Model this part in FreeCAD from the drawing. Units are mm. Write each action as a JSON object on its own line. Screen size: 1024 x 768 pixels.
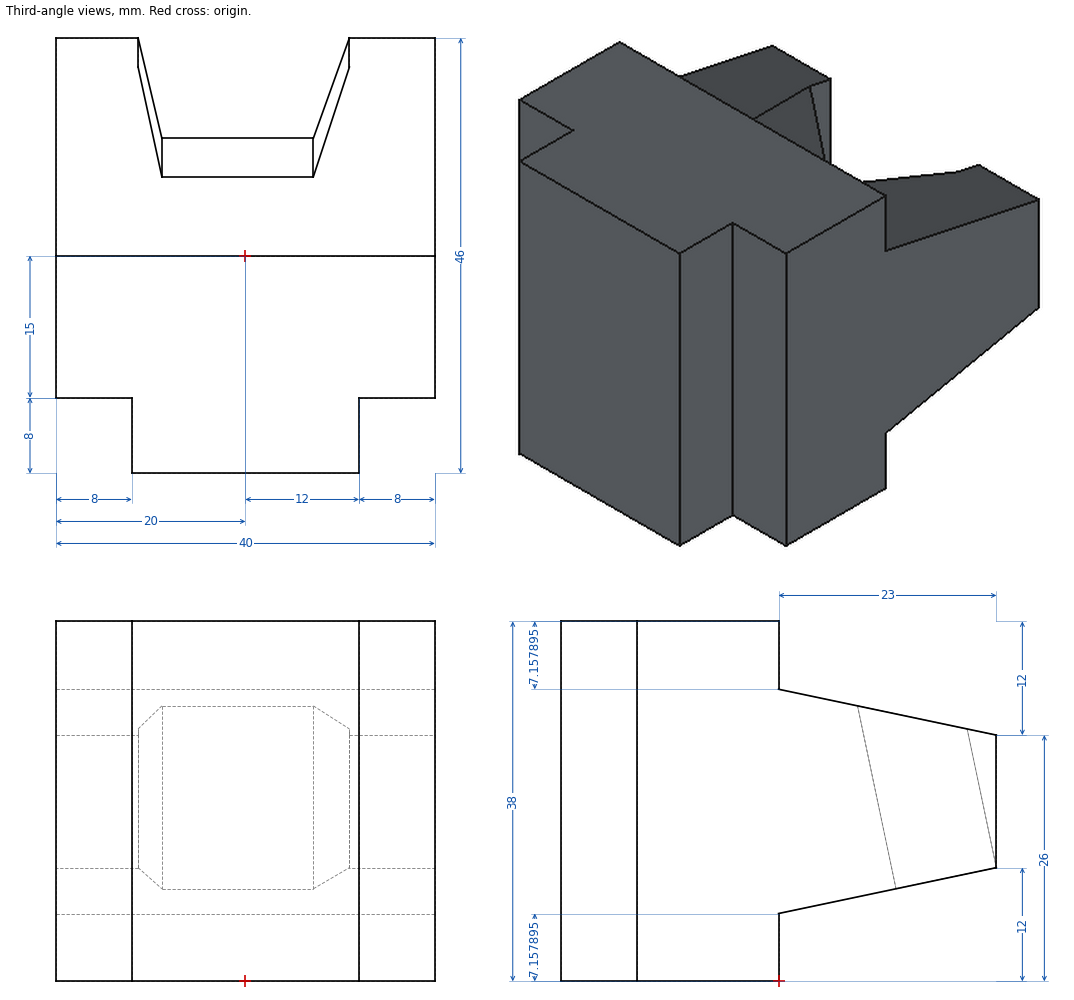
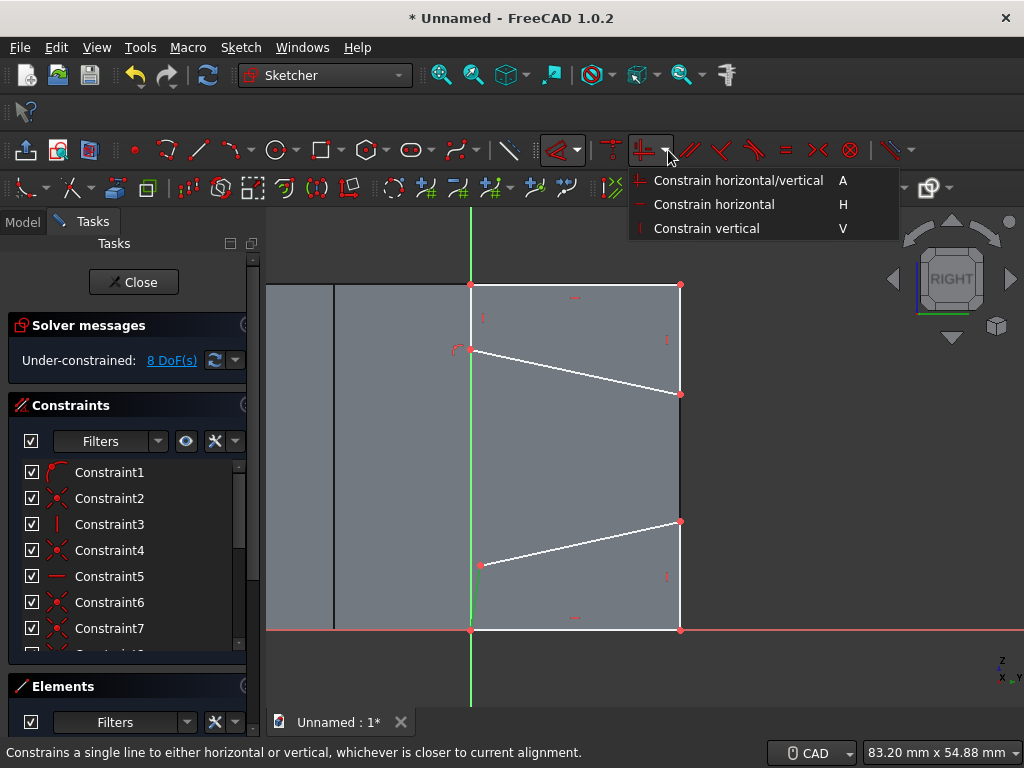
{"action": "left_click", "coordinate": [764, 228]}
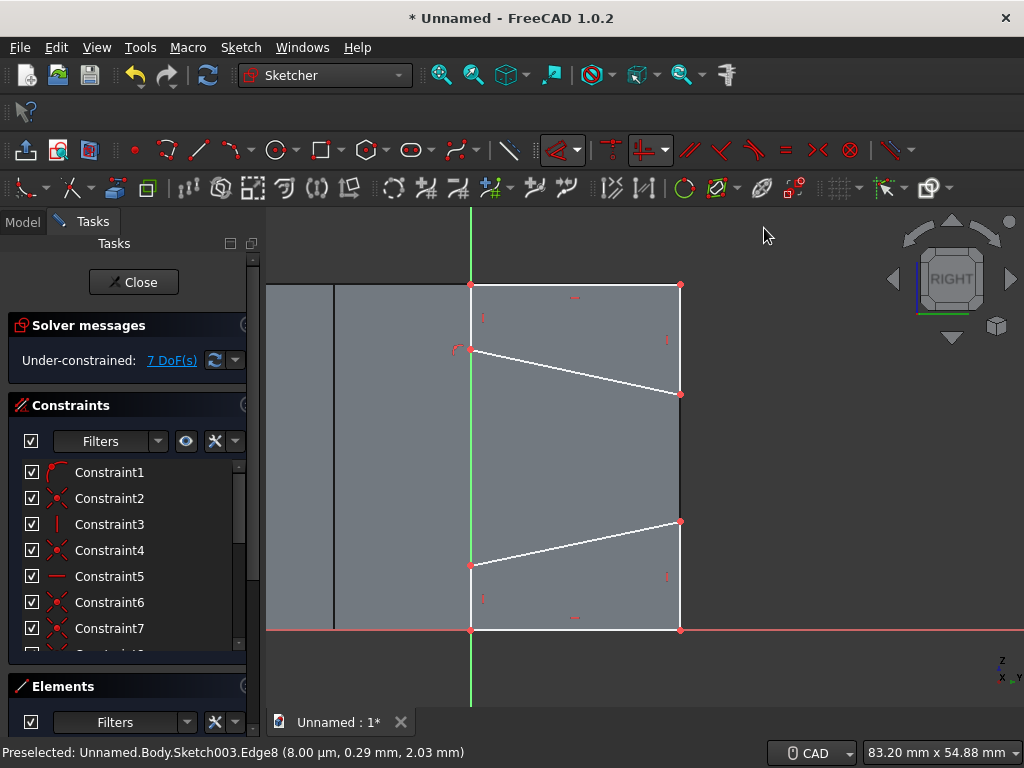
{"action": "left_click", "coordinate": [680, 362]}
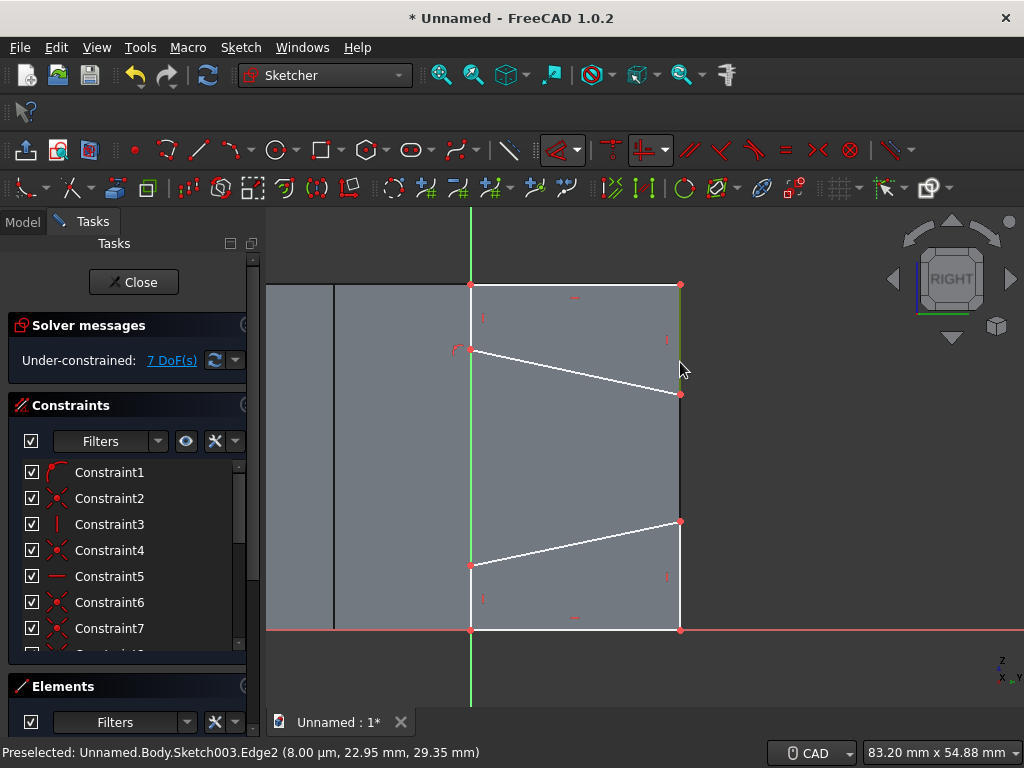
{"action": "key", "text": "i"}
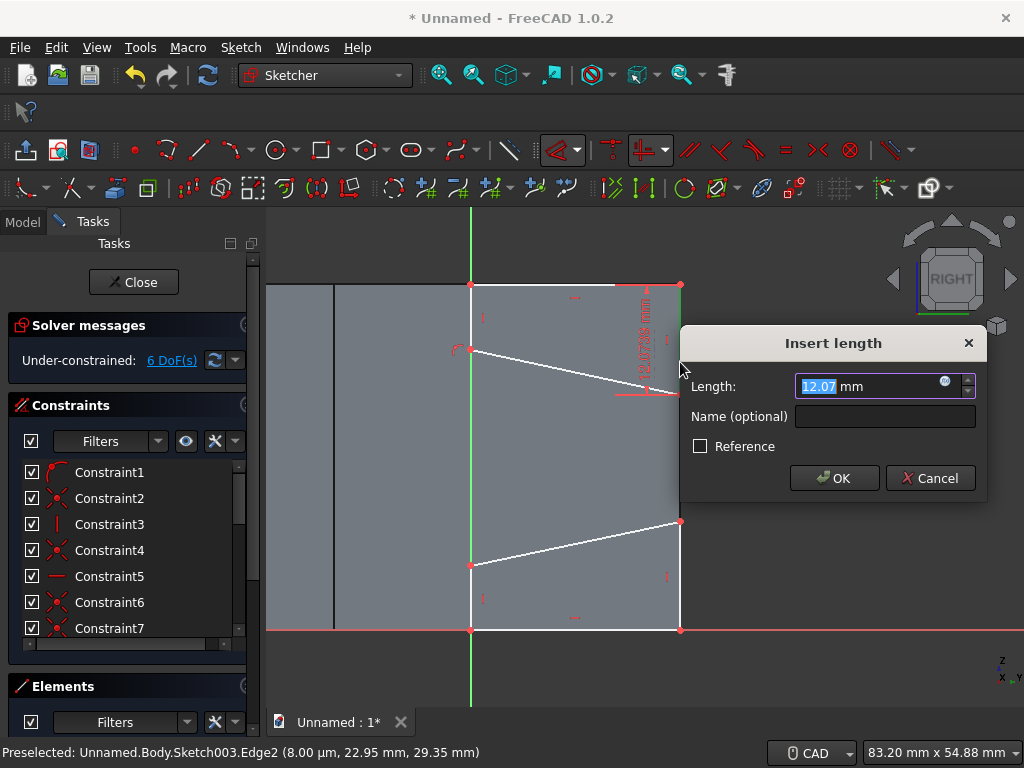
{"action": "type", "text": "12"}
{"action": "key", "text": "Return"}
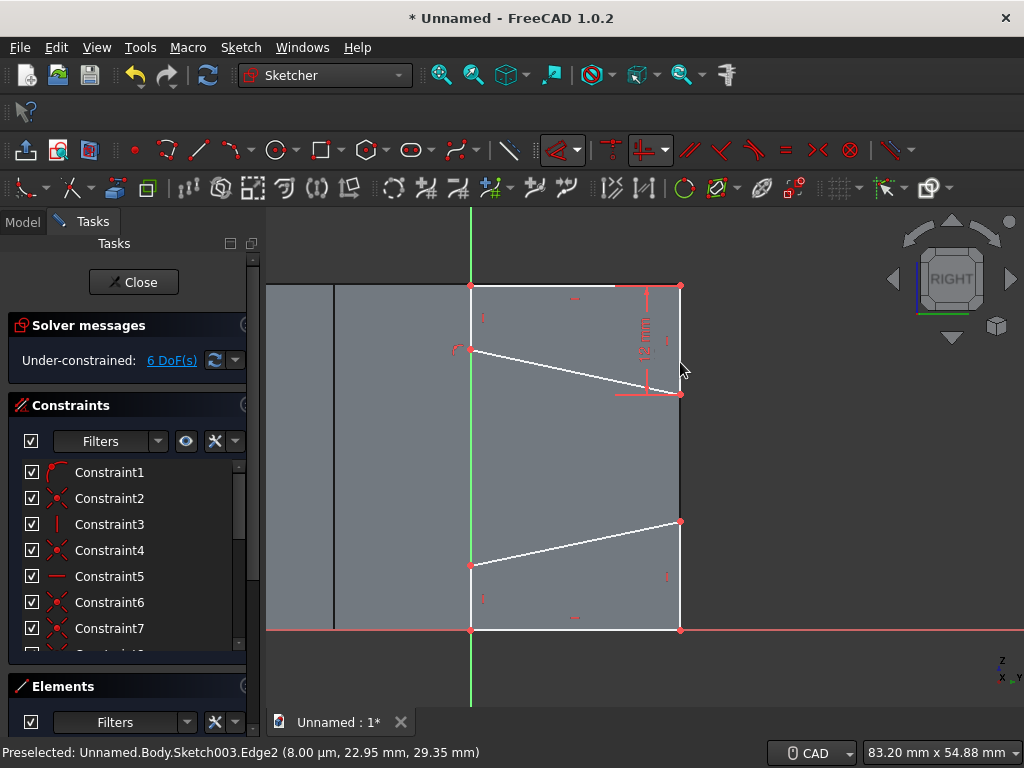
{"action": "left_click", "coordinate": [617, 286]}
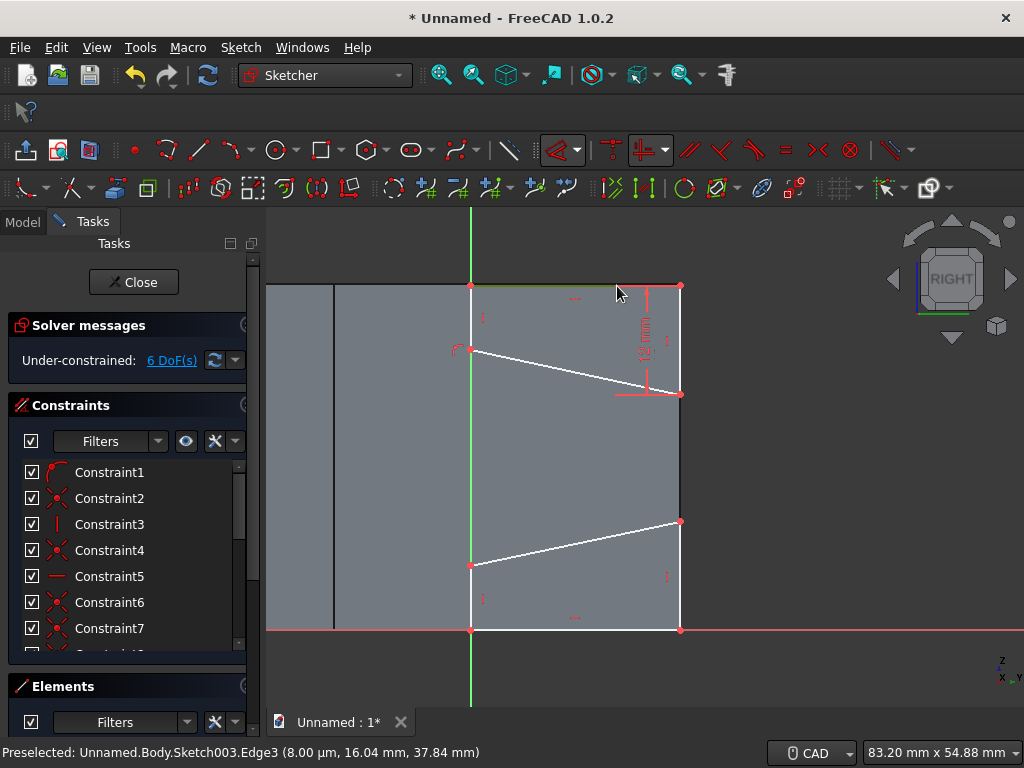
{"action": "left_click", "coordinate": [580, 150]}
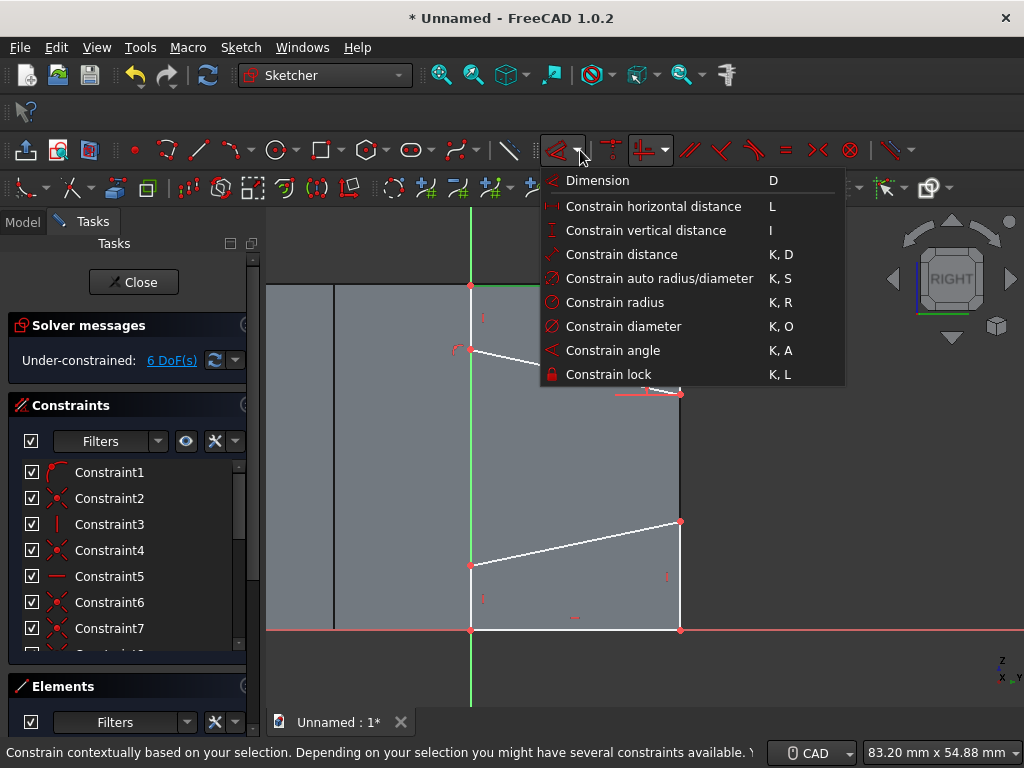
{"action": "left_click", "coordinate": [693, 206]}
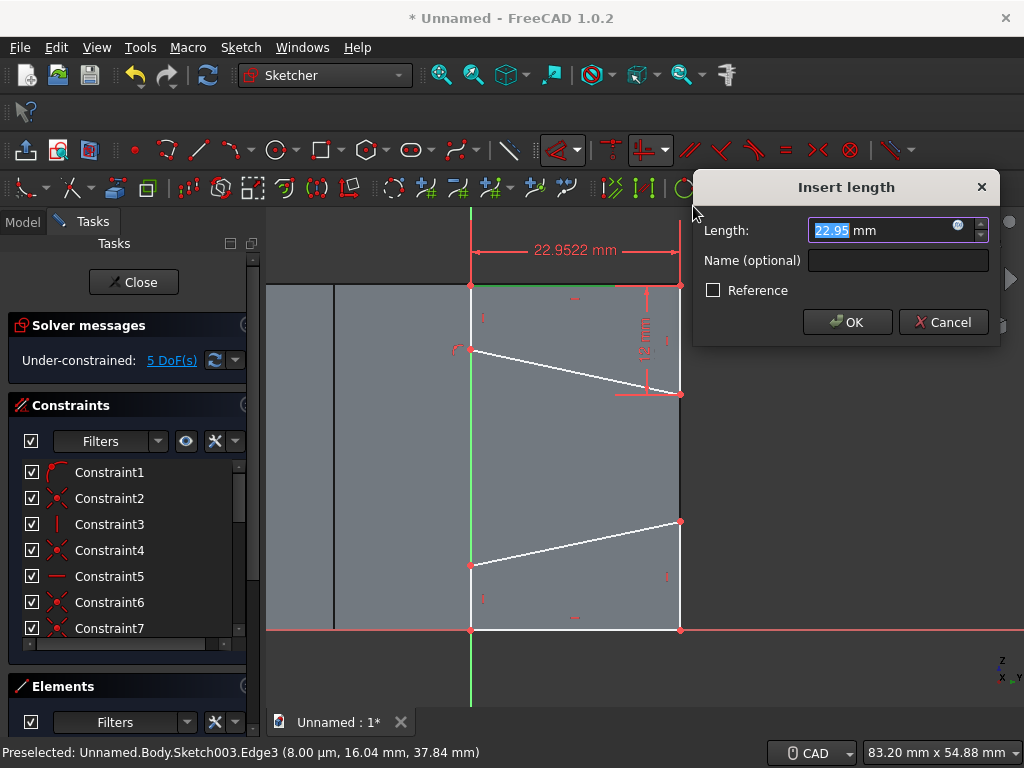
{"action": "type", "text": "23"}
{"action": "key", "text": "Return"}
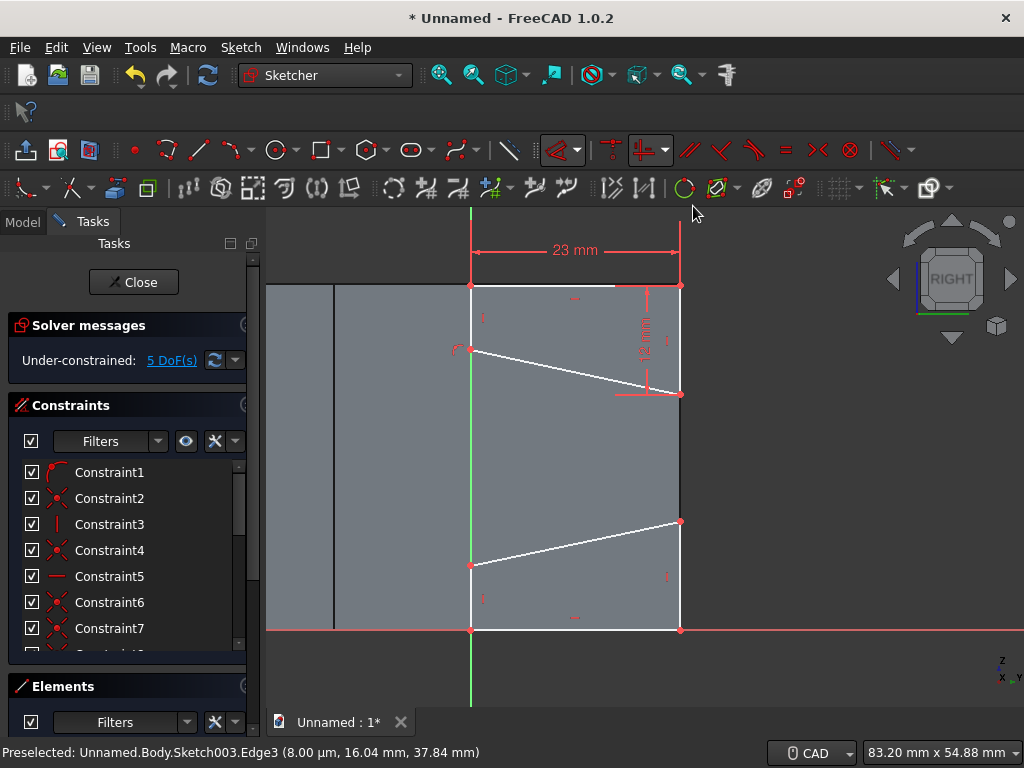
{"action": "left_click", "coordinate": [534, 630]}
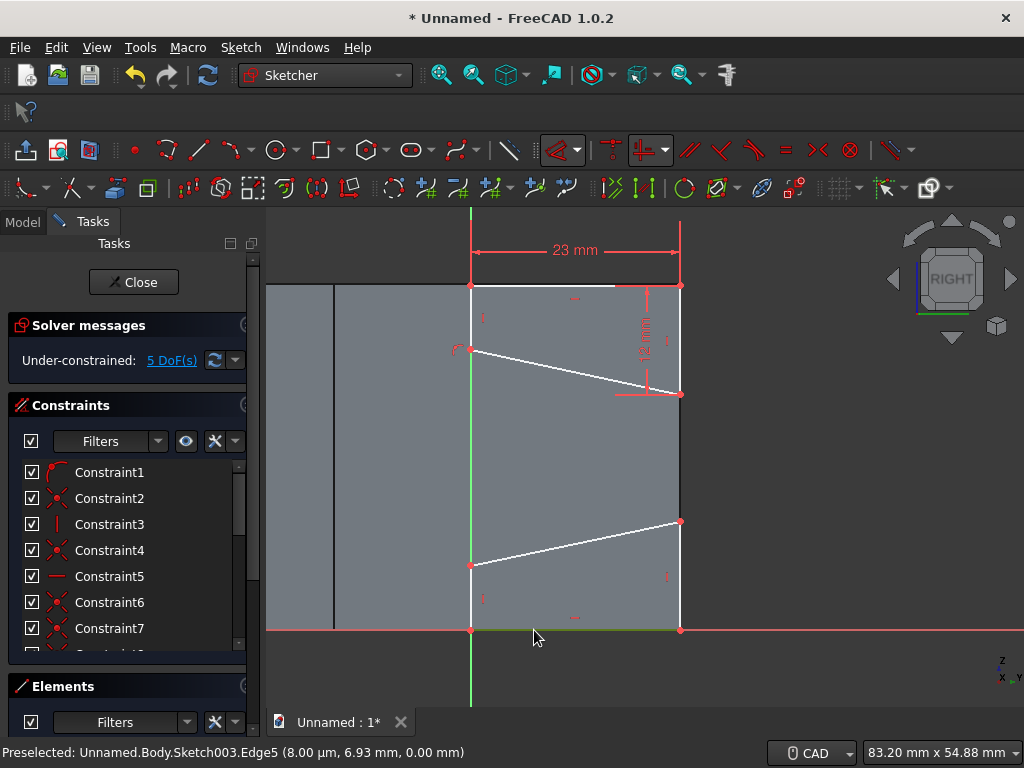
{"action": "left_click", "coordinate": [580, 150]}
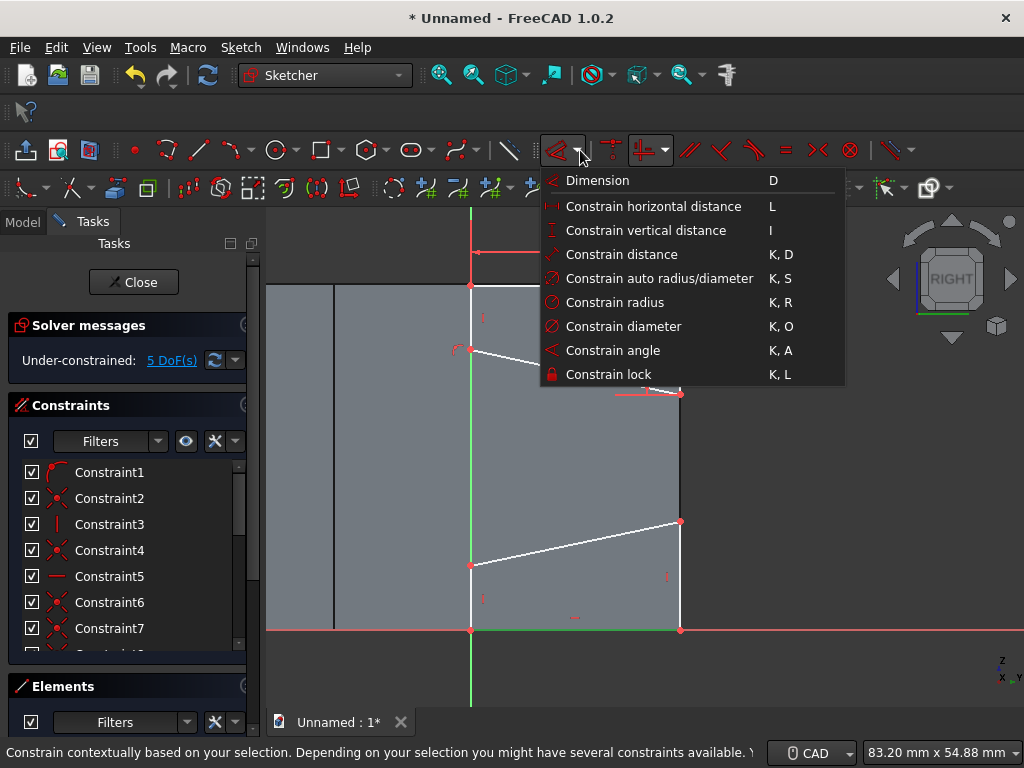
{"action": "left_click", "coordinate": [693, 206]}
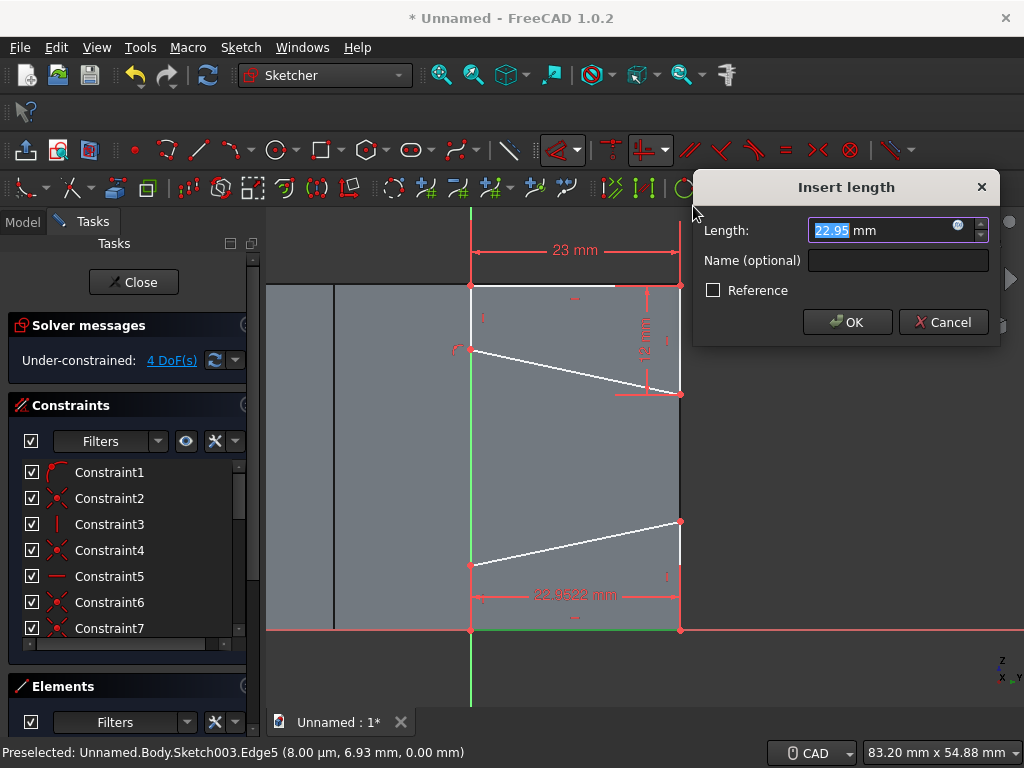
{"action": "type", "text": "23"}
{"action": "key", "text": "Return"}